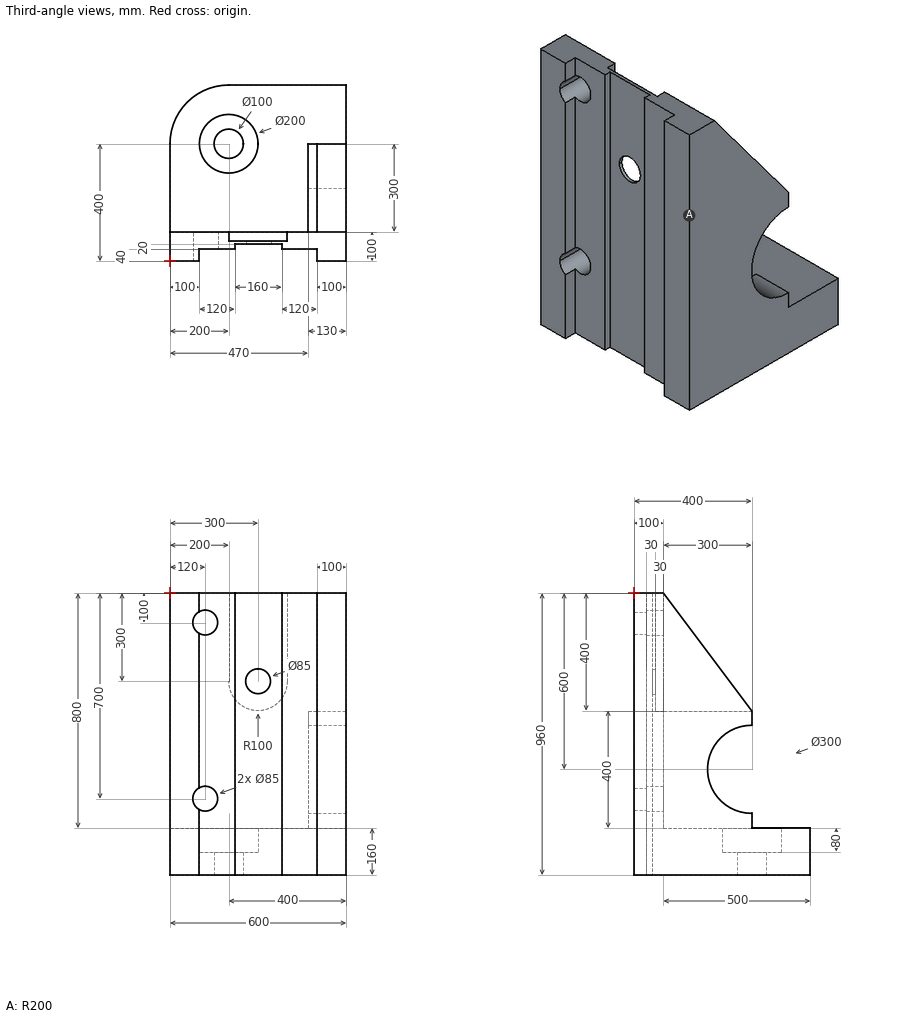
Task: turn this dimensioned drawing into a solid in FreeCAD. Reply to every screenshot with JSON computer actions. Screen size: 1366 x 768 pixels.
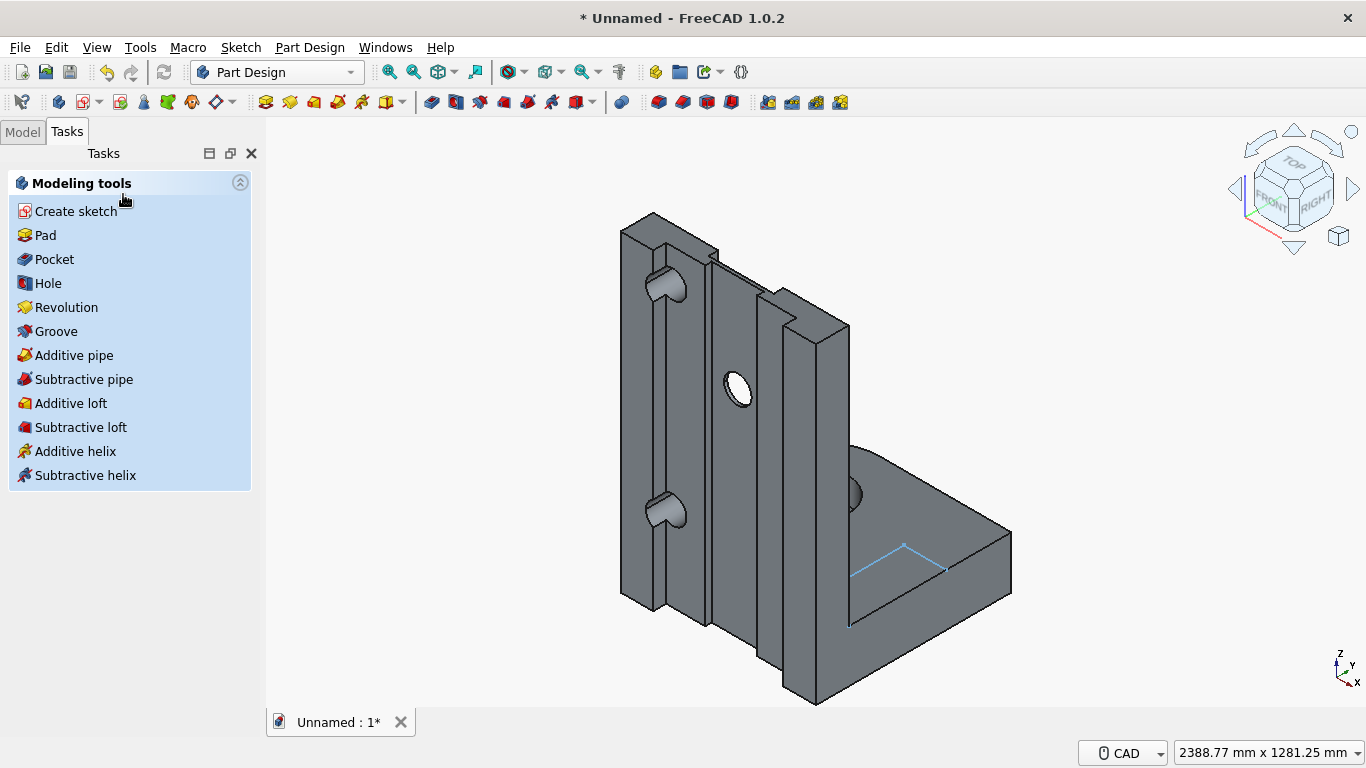
{"action": "left_click", "coordinate": [266, 102]}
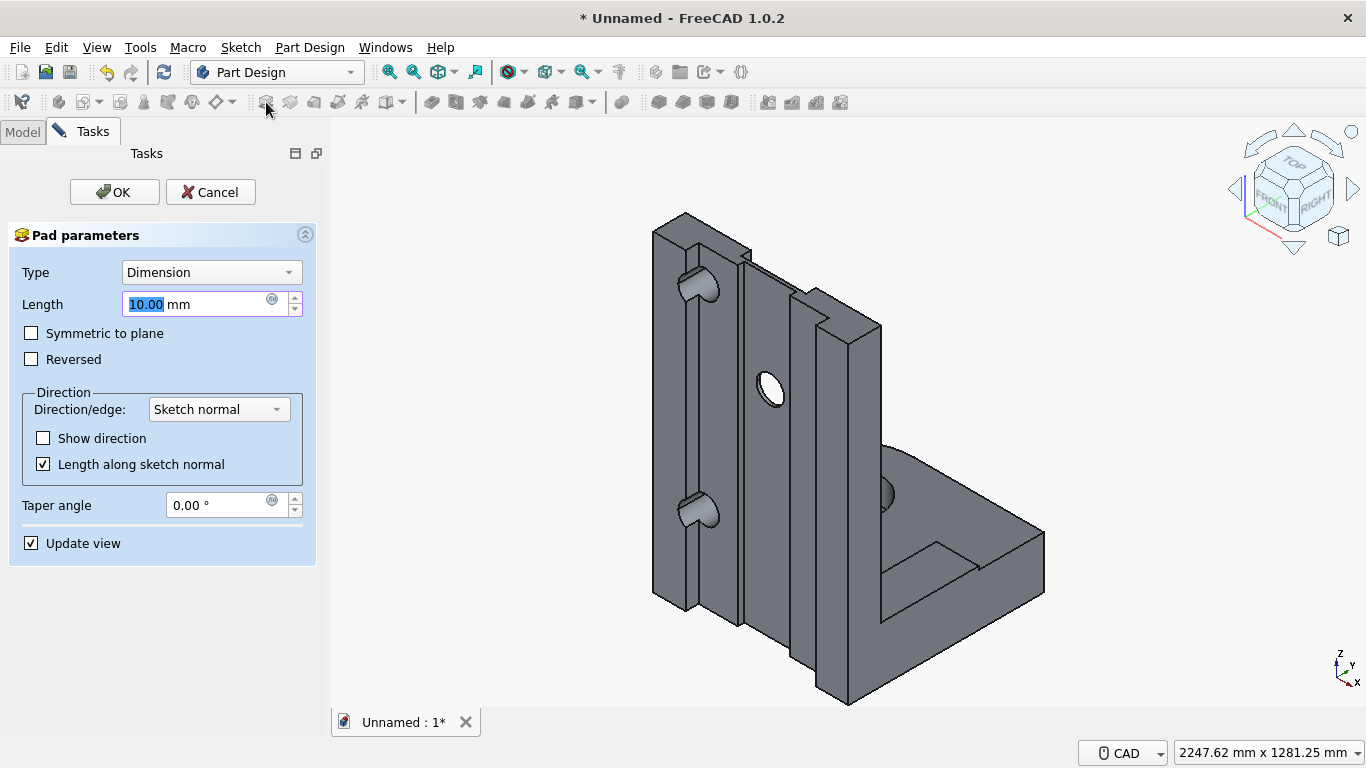
{"action": "type", "text": "400"}
{"action": "key", "text": "Tab"}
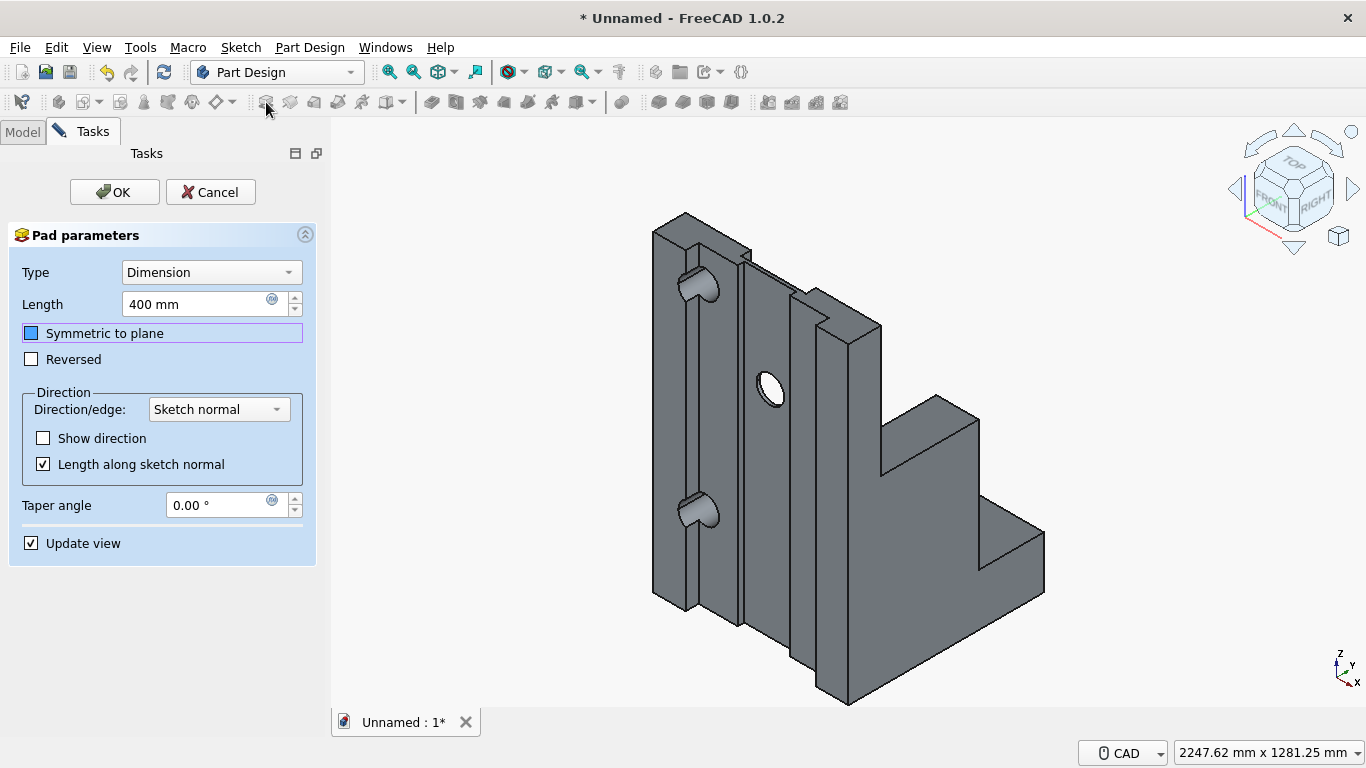
{"action": "left_click", "coordinate": [115, 192]}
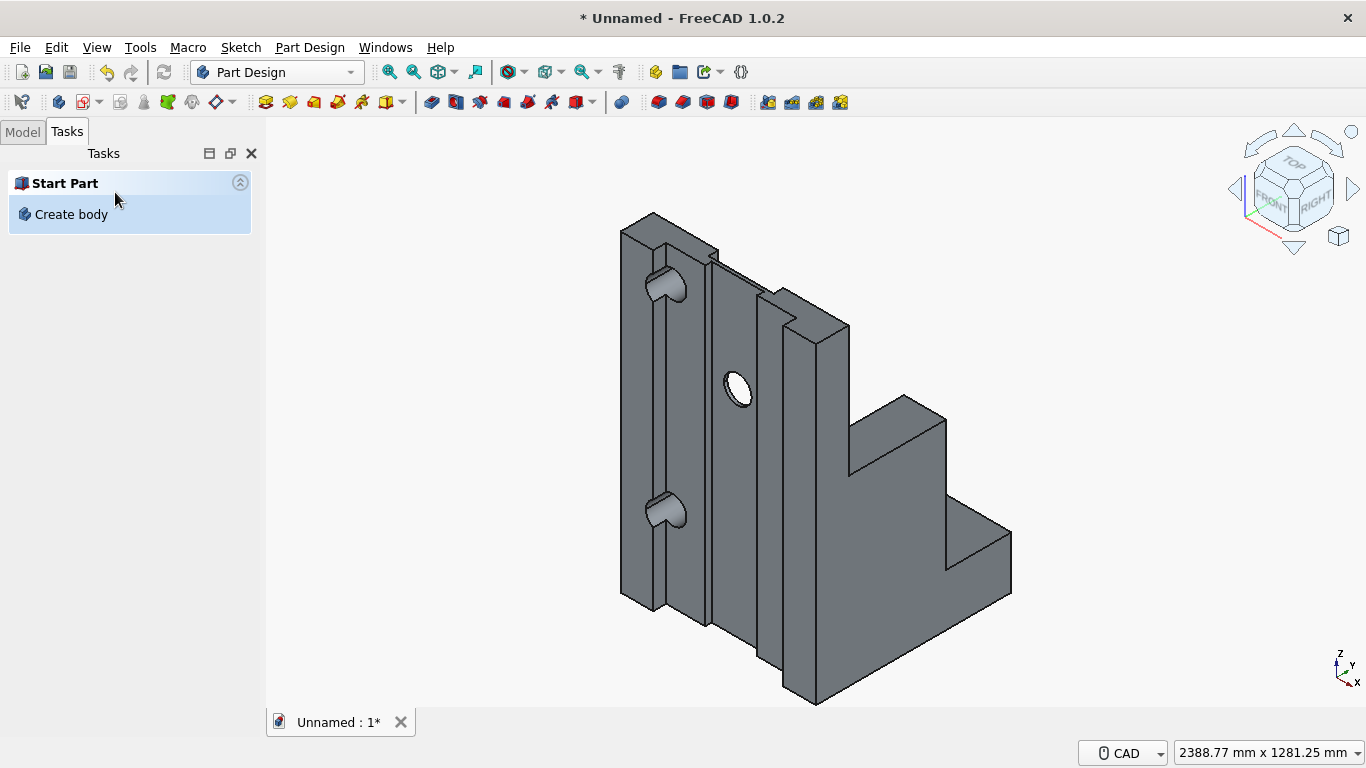
{"action": "left_click", "coordinate": [886, 535]}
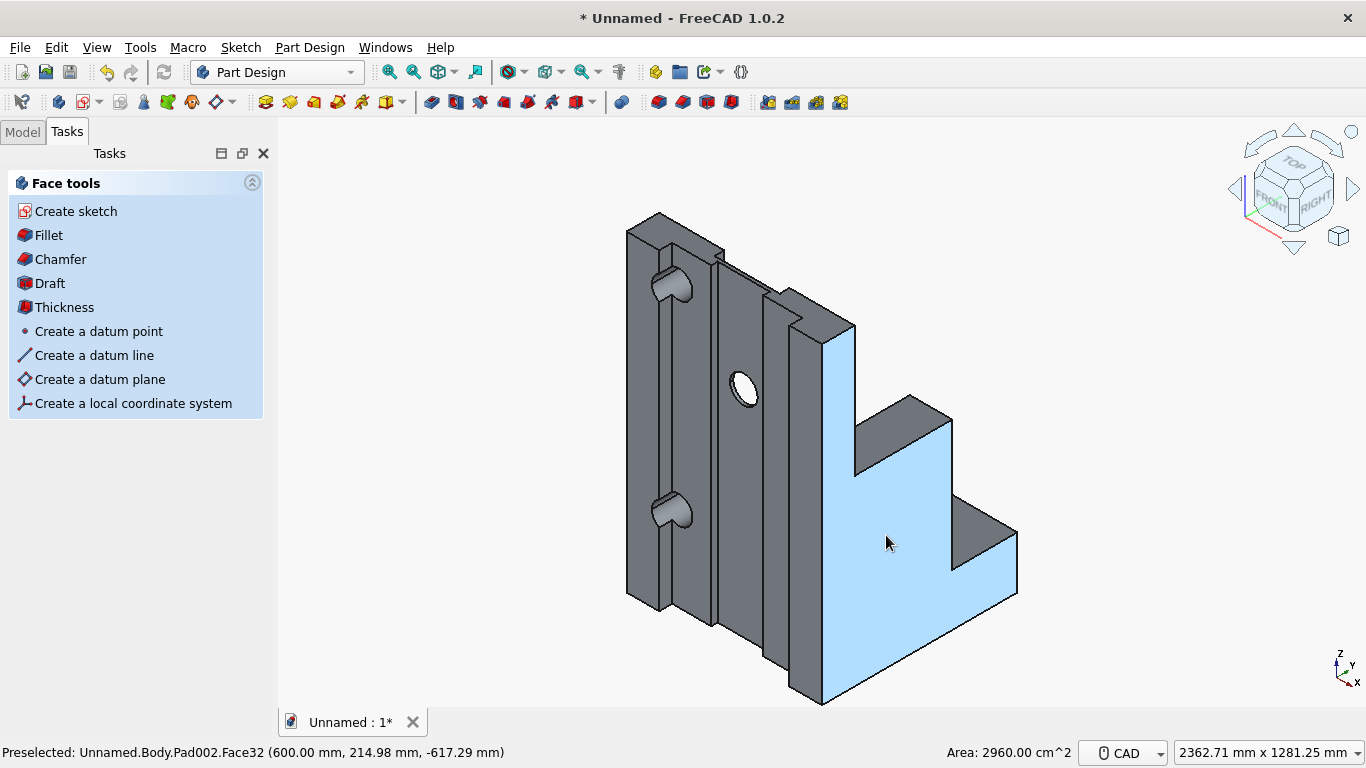
{"action": "left_click", "coordinate": [84, 102]}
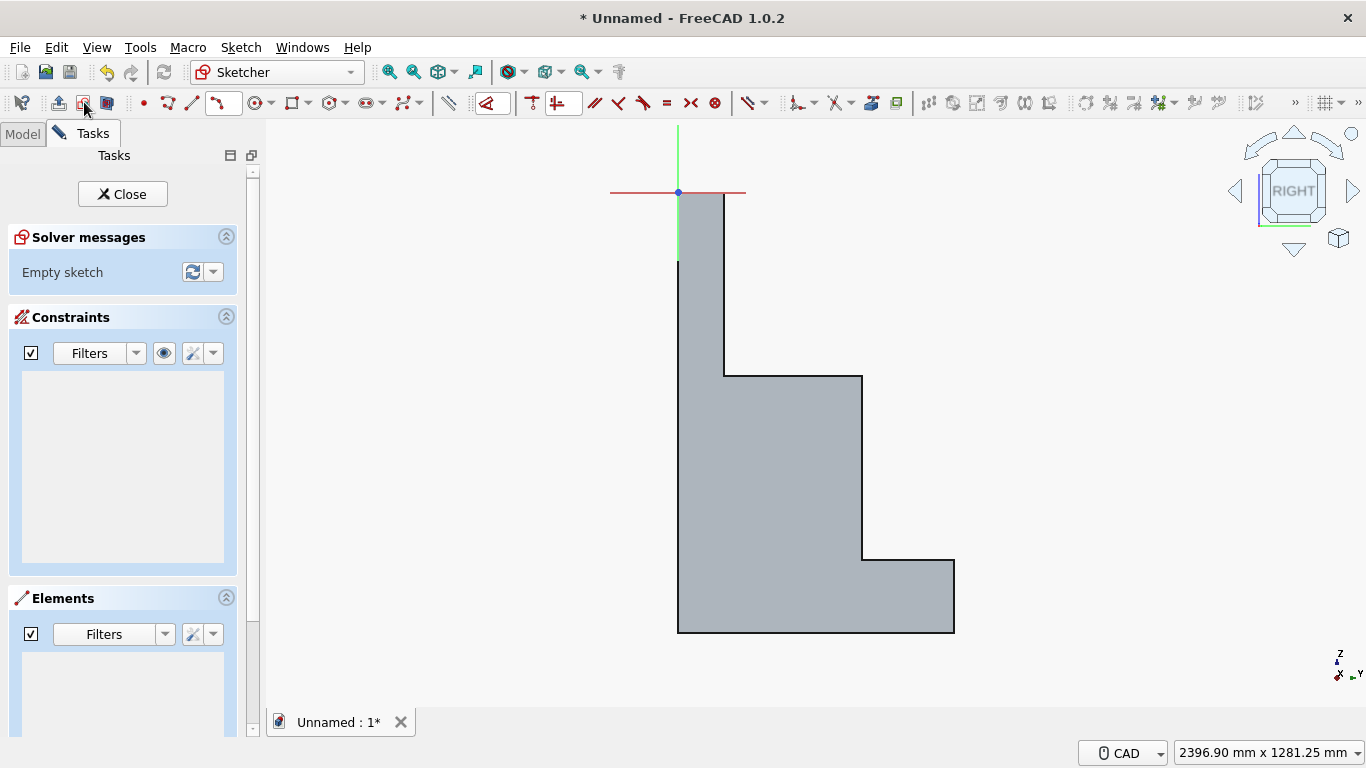
{"action": "scroll", "coordinate": [928, 500], "scroll_direction": "up", "scroll_amount": 5}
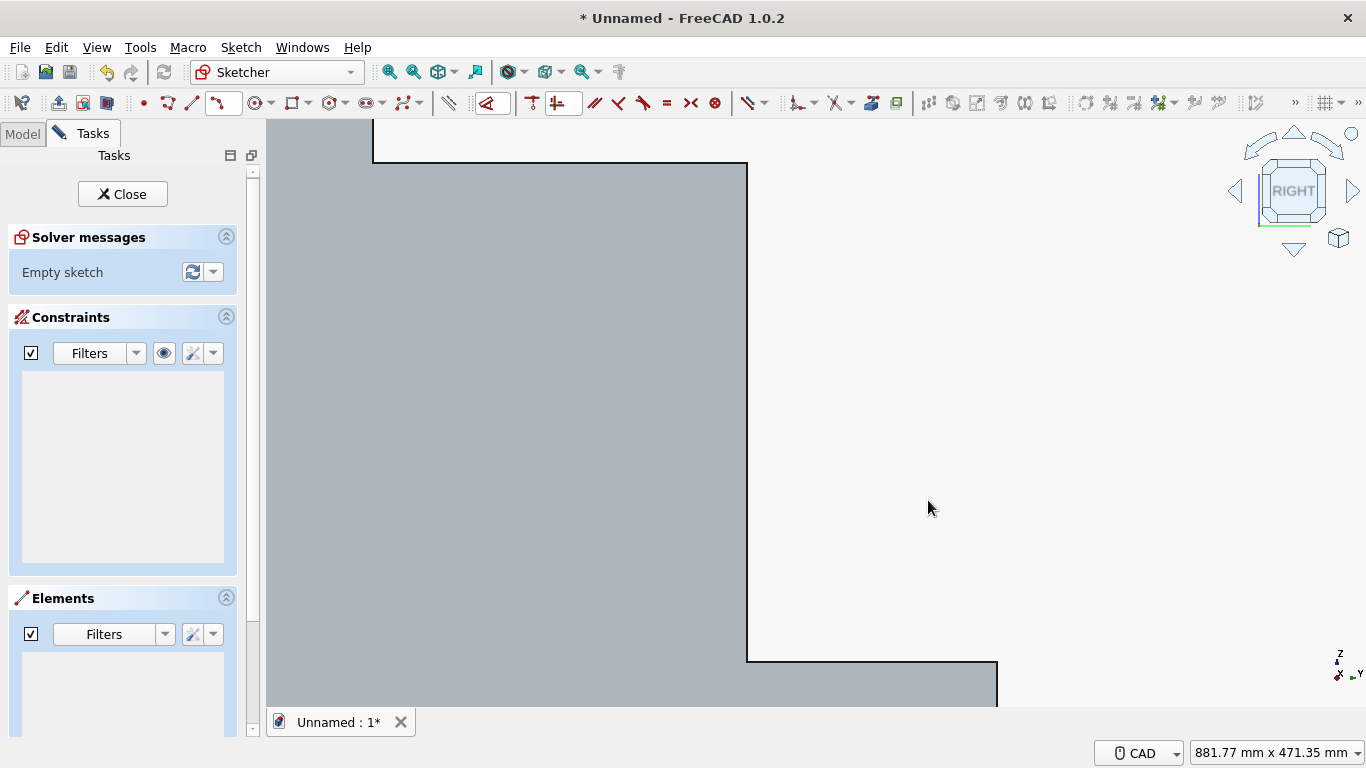
{"action": "left_click", "coordinate": [256, 104]}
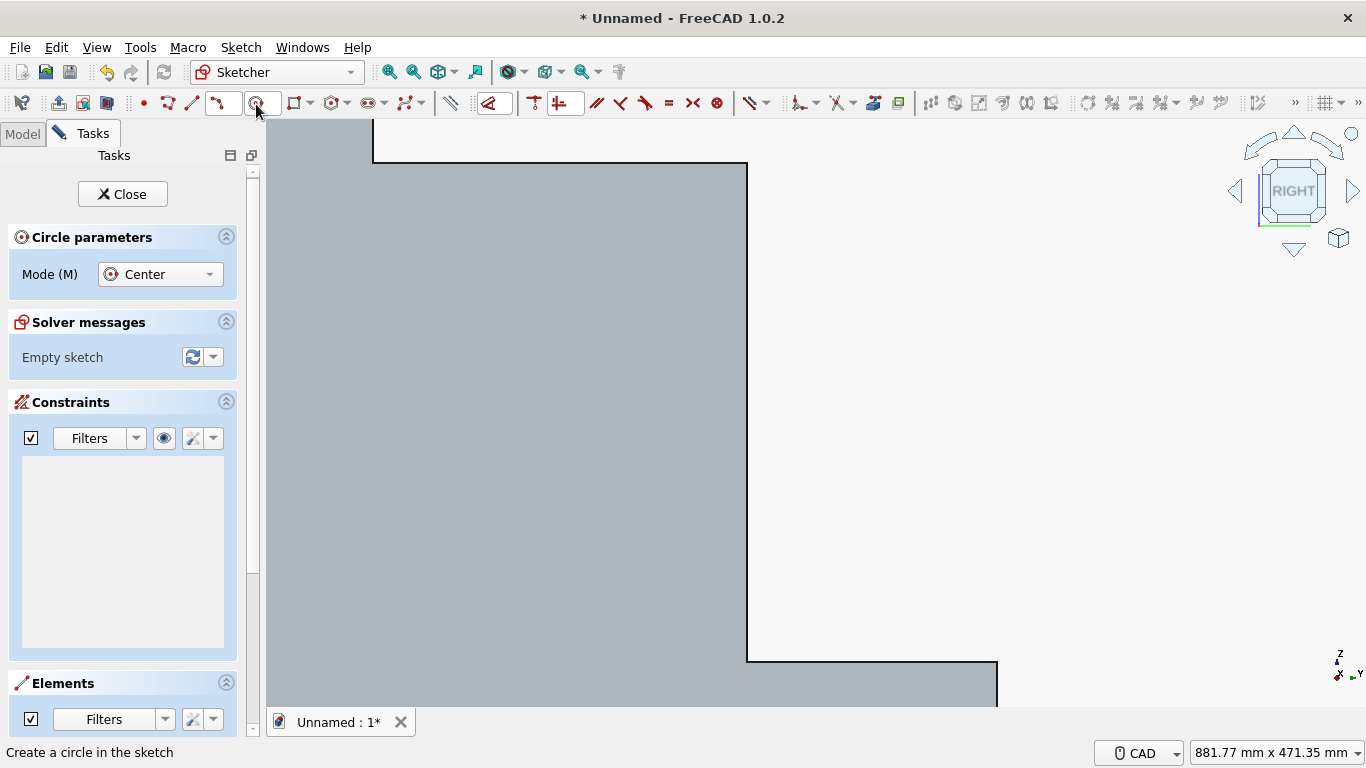
{"action": "left_click", "coordinate": [747, 412]}
{"action": "left_click", "coordinate": [880, 280]}
{"action": "key", "text": "Escape"}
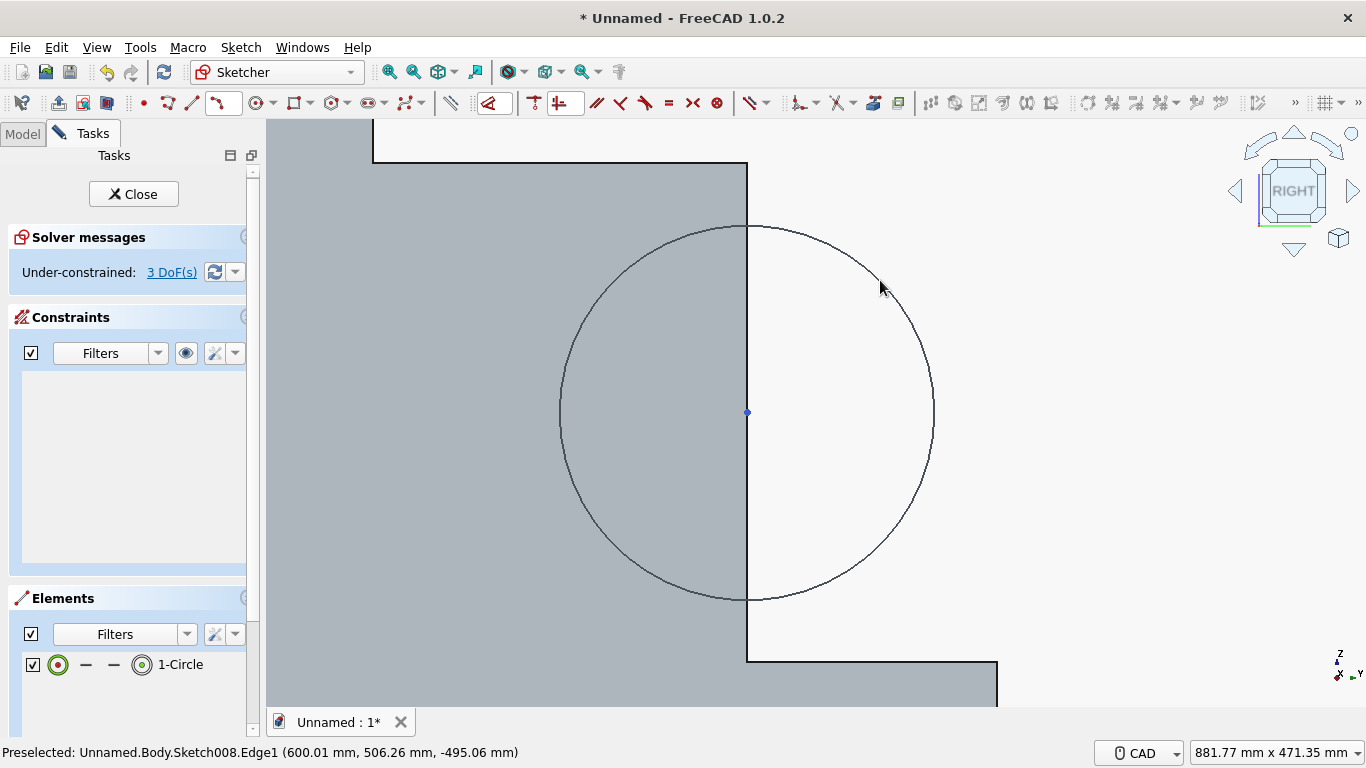
{"action": "left_click", "coordinate": [879, 280]}